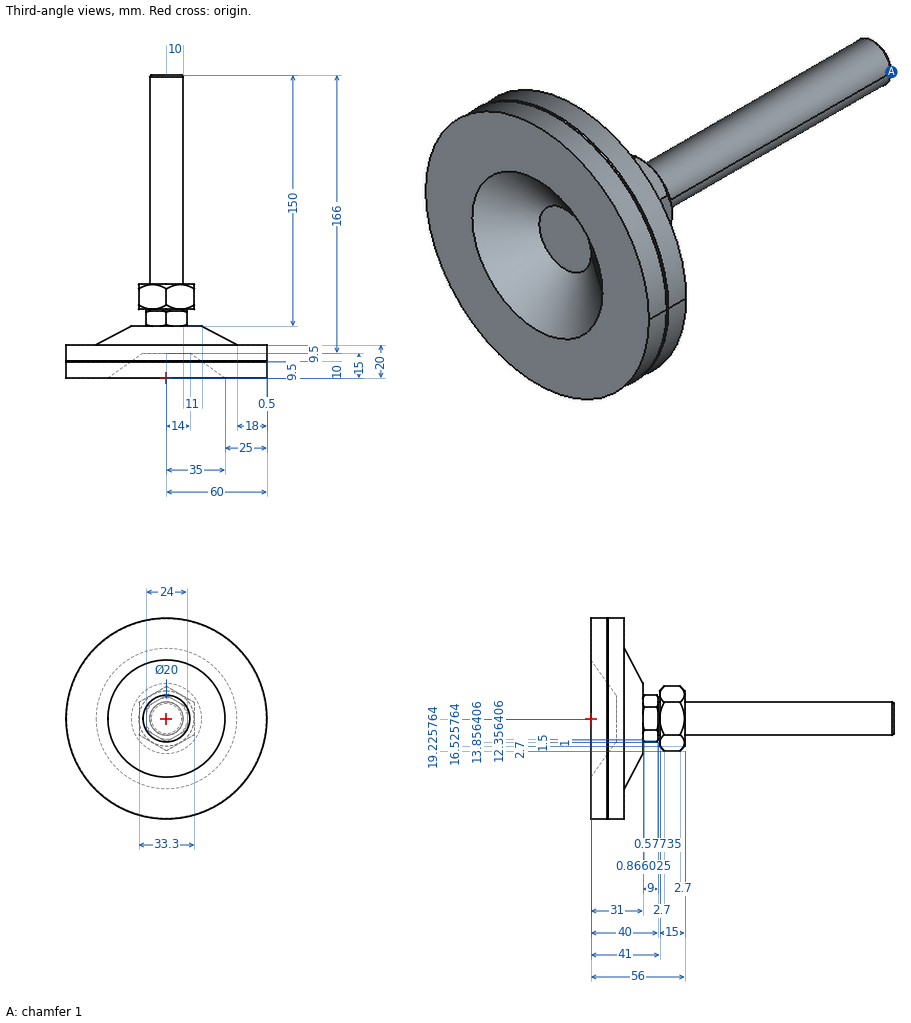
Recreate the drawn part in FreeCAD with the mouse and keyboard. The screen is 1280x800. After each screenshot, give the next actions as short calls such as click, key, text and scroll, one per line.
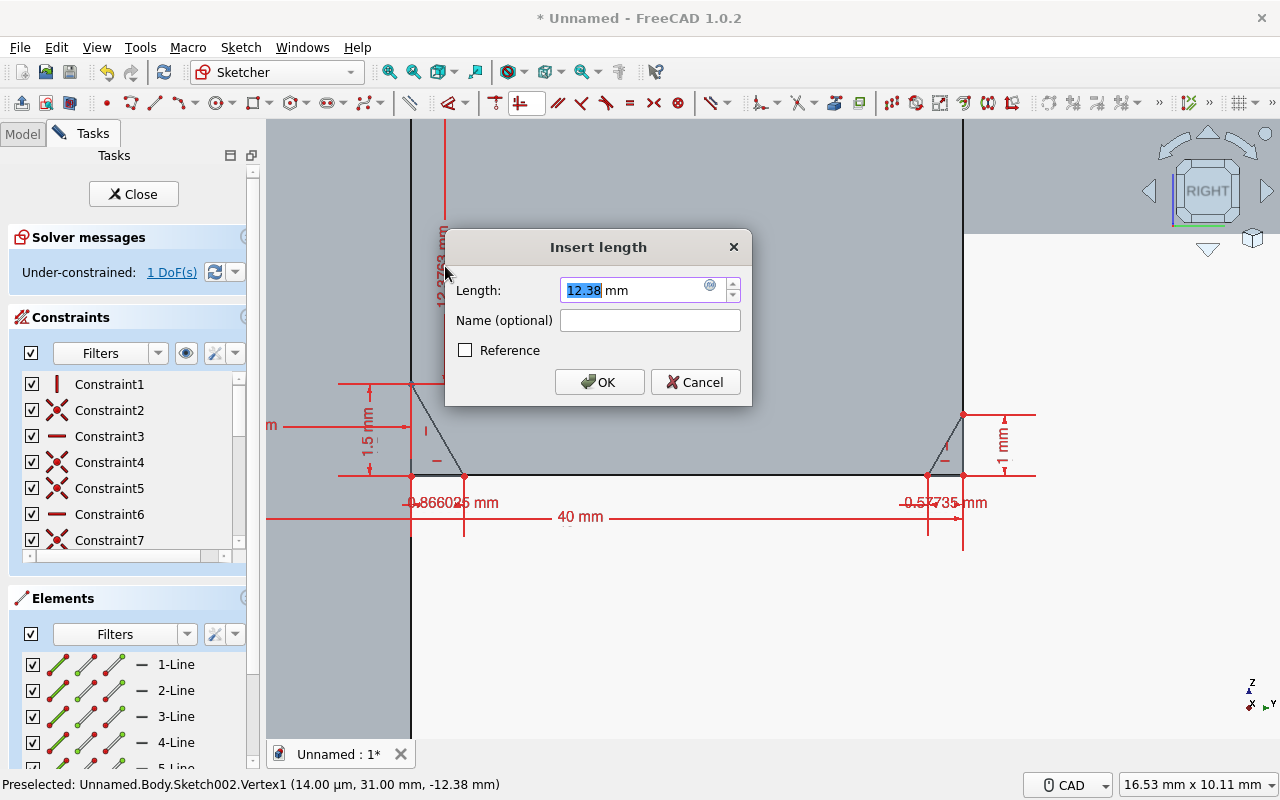
text(12.356406)
key(Return)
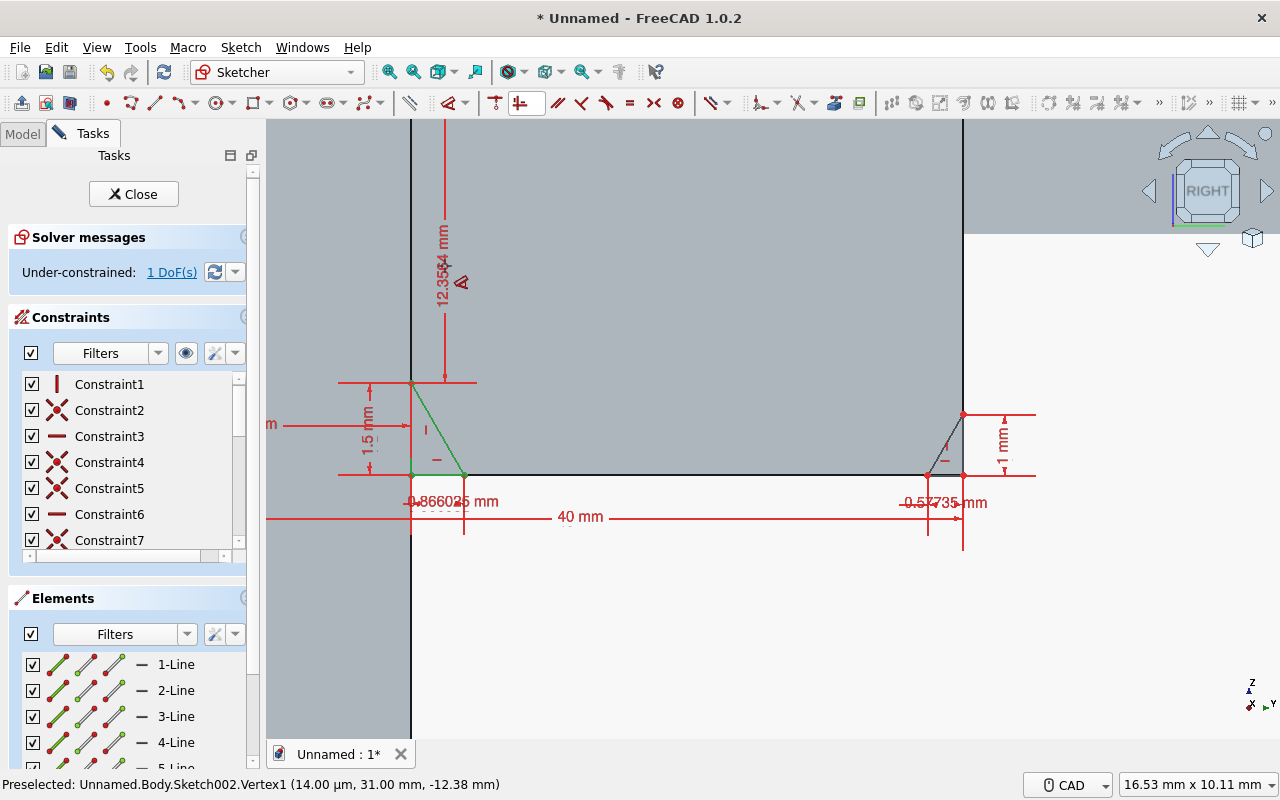
click(928, 476)
click(962, 311)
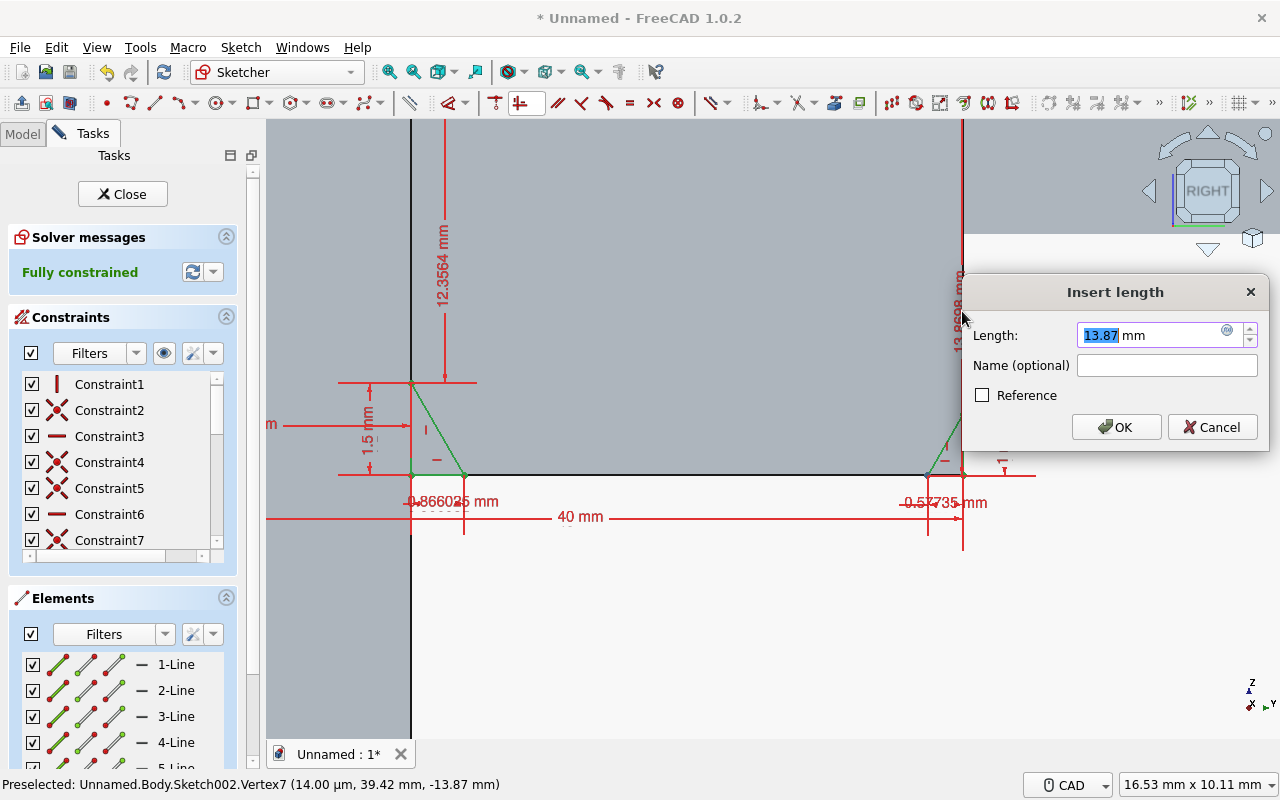
text(13.856406)
key(Return)
key(Escape)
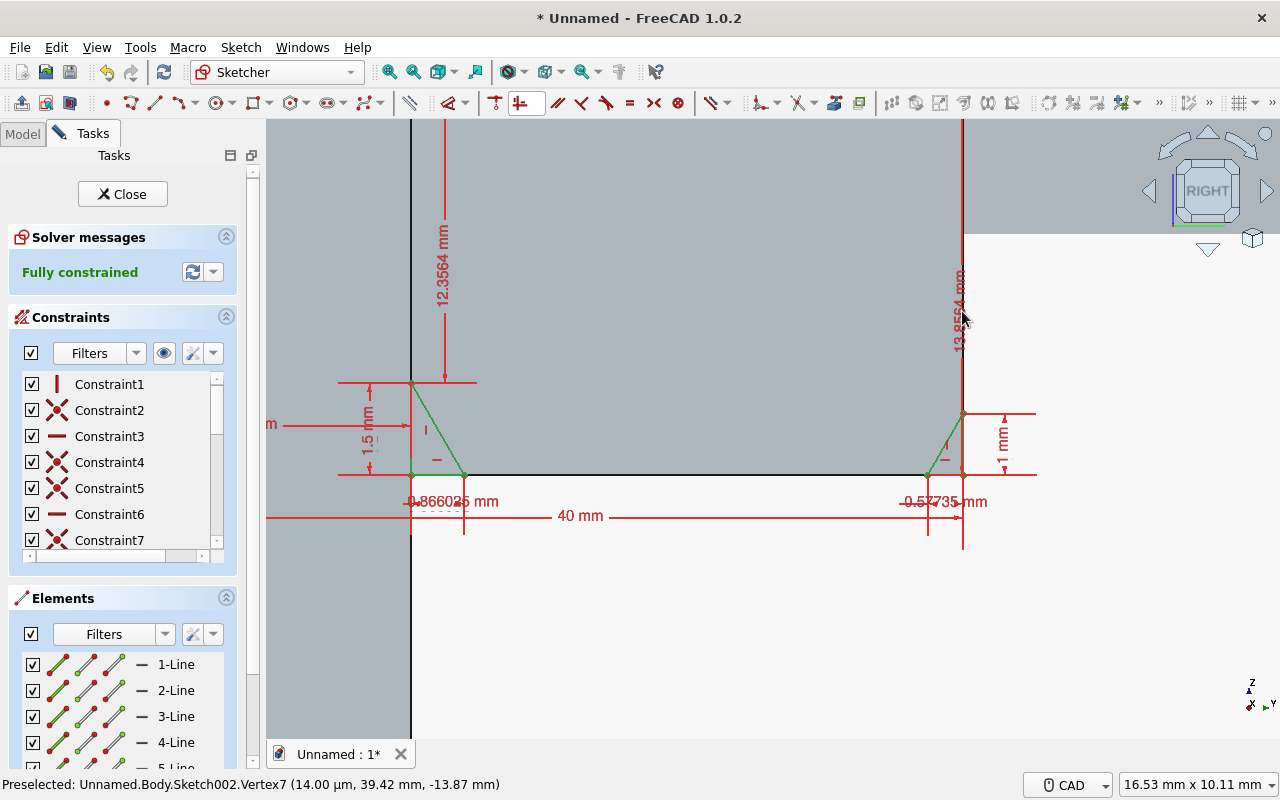
click(123, 194)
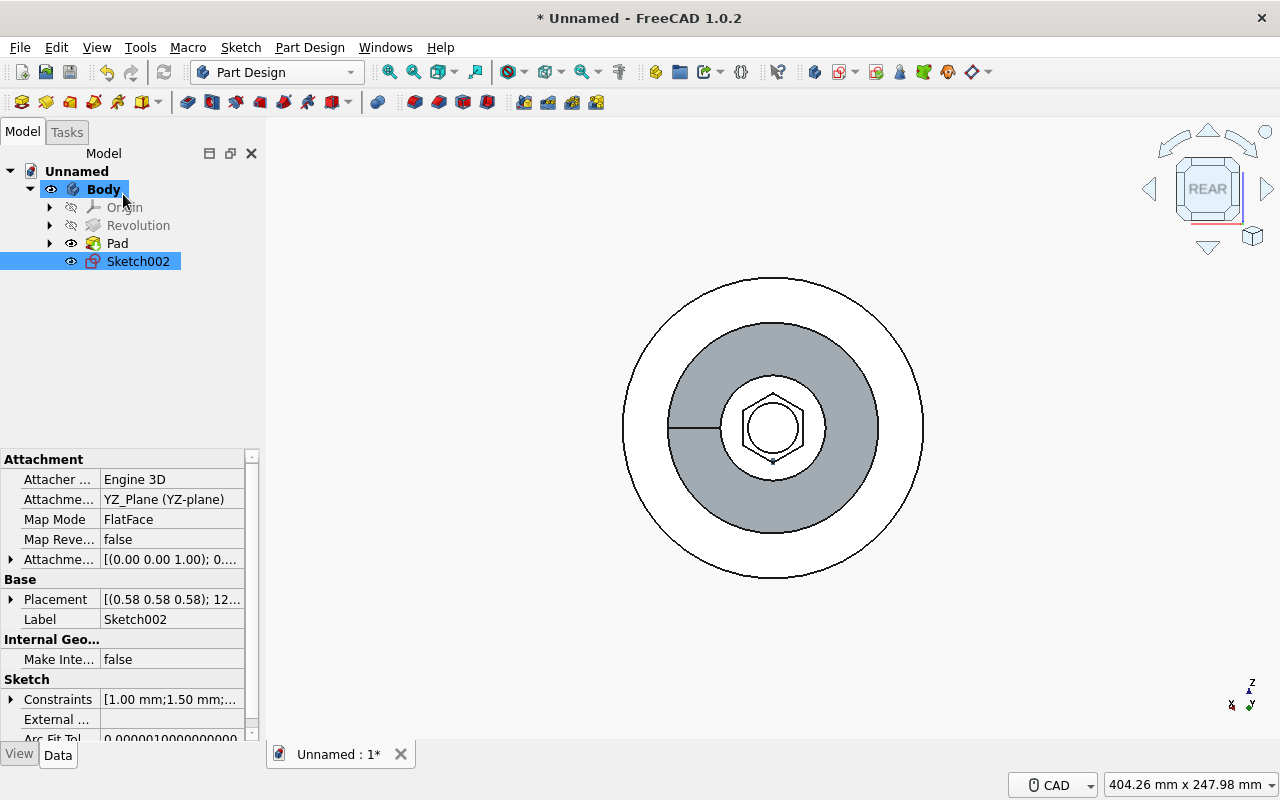
click(236, 102)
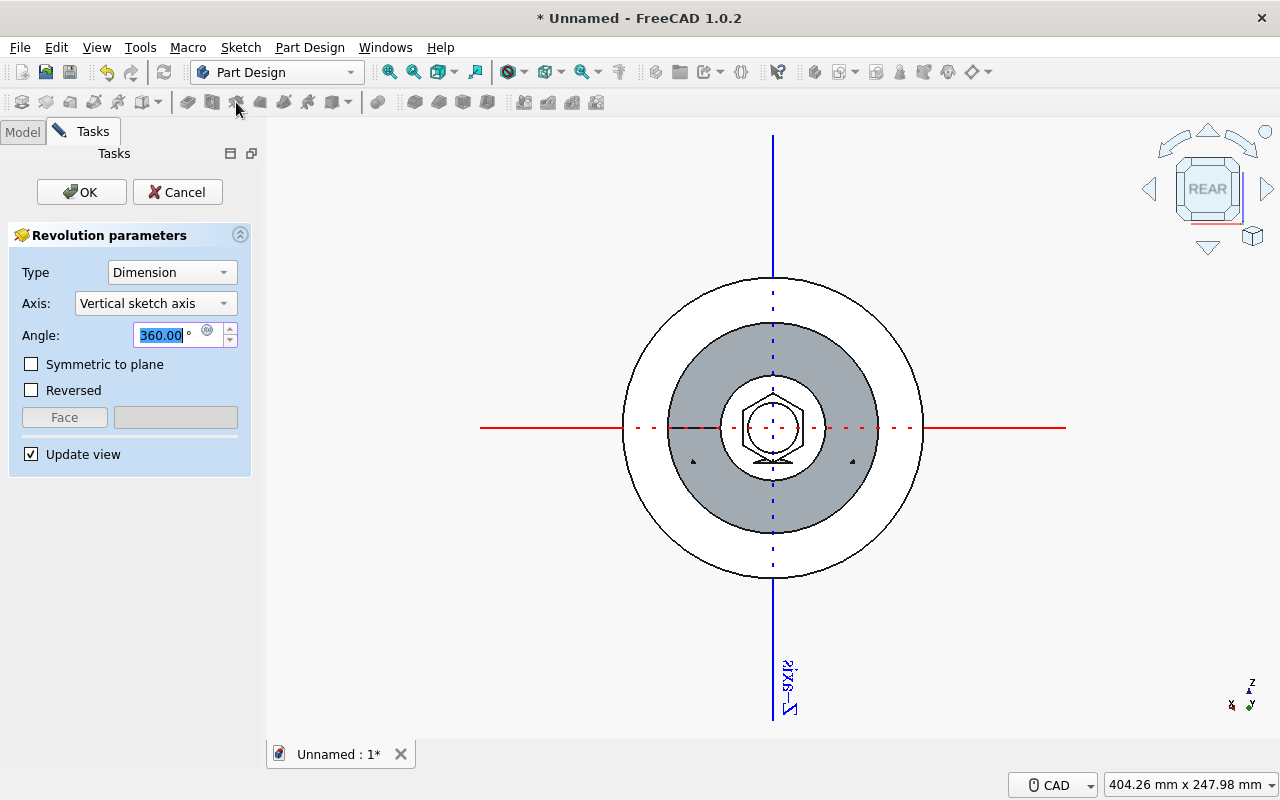
click(156, 304)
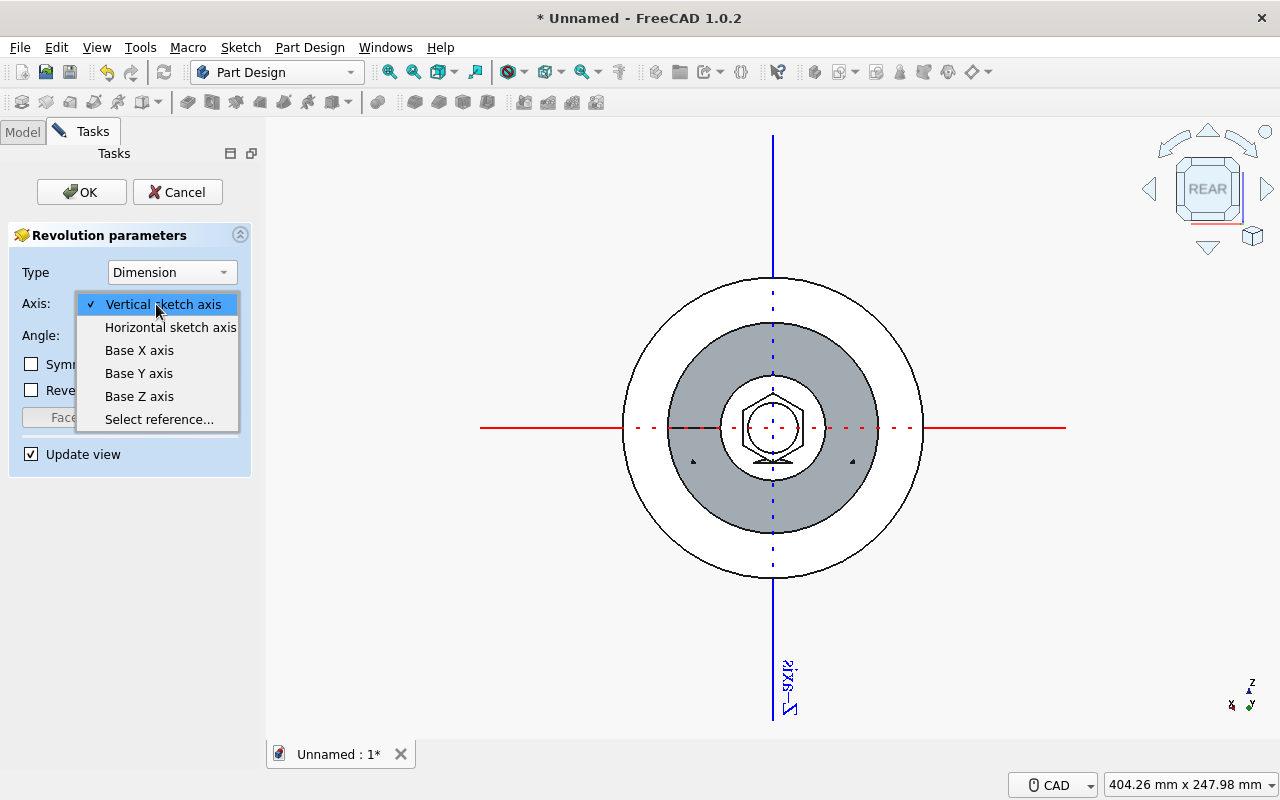
click(156, 328)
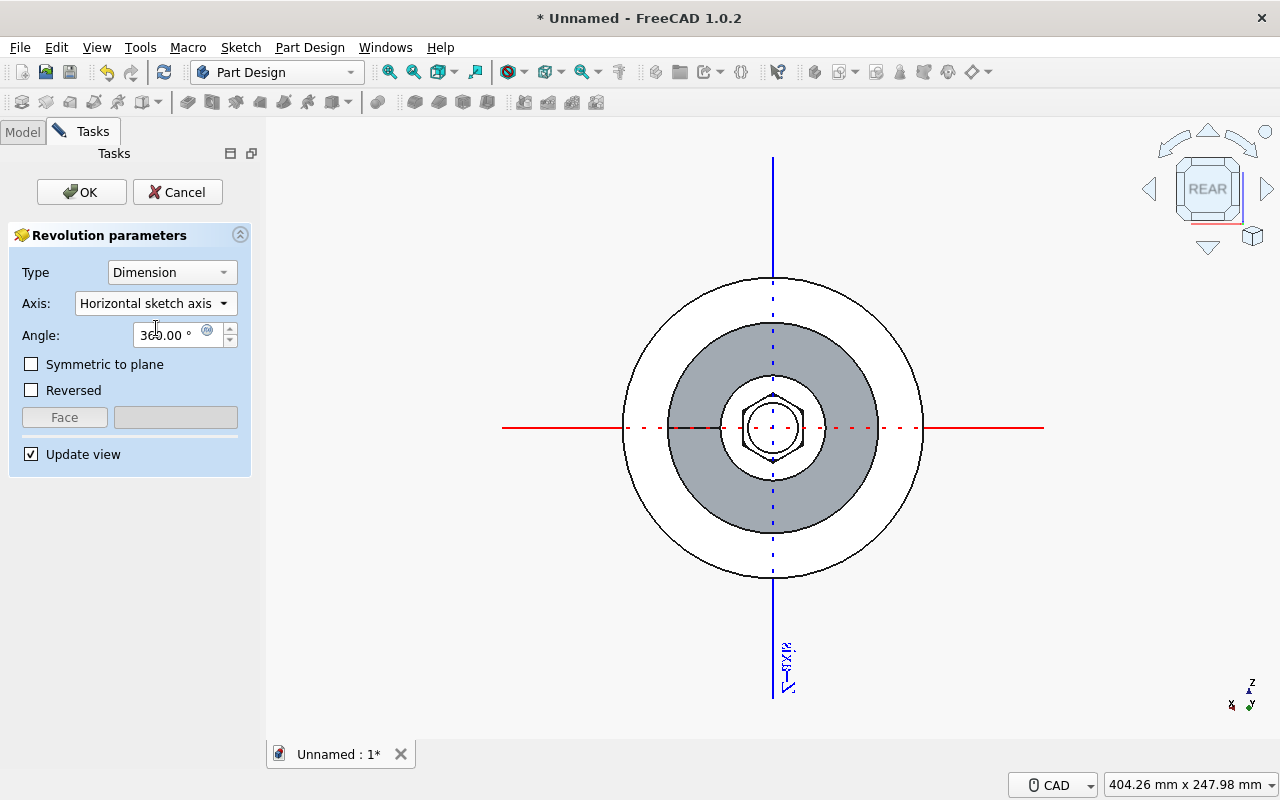
click(82, 192)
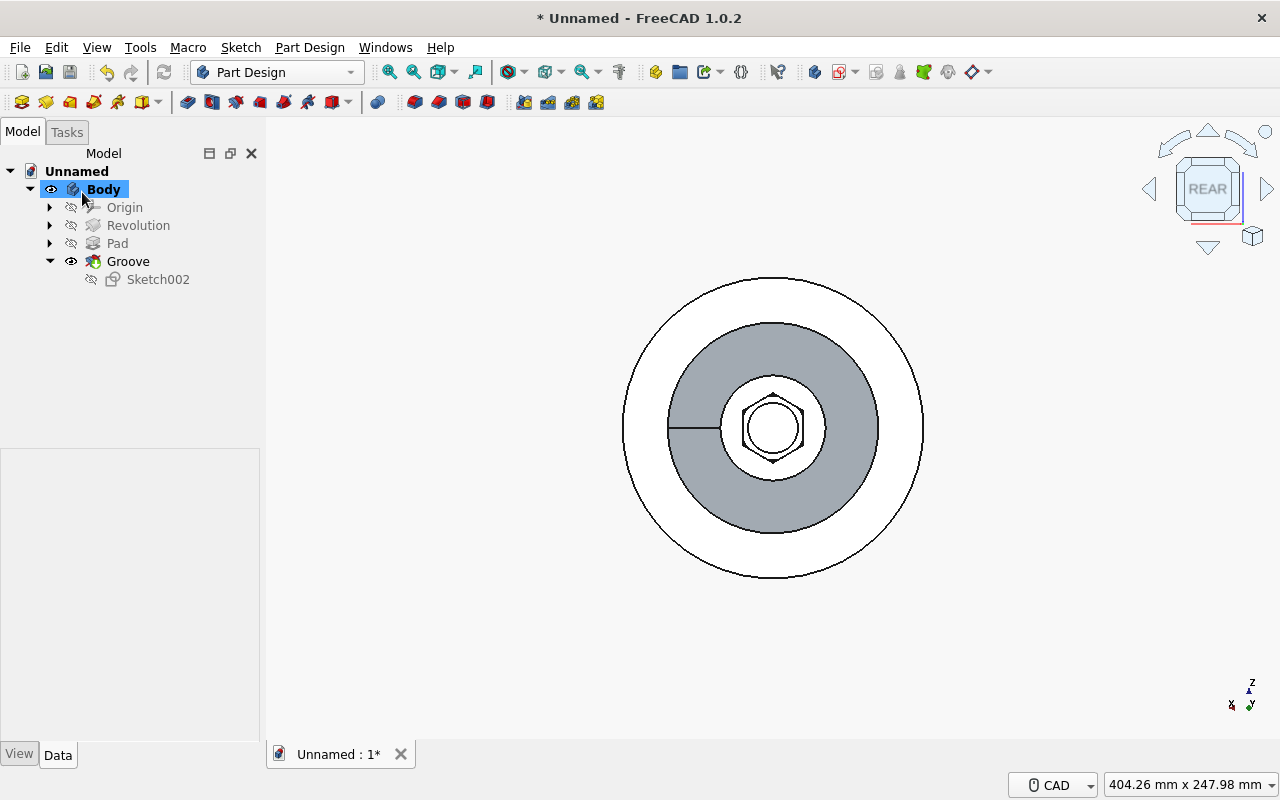
click(50, 207)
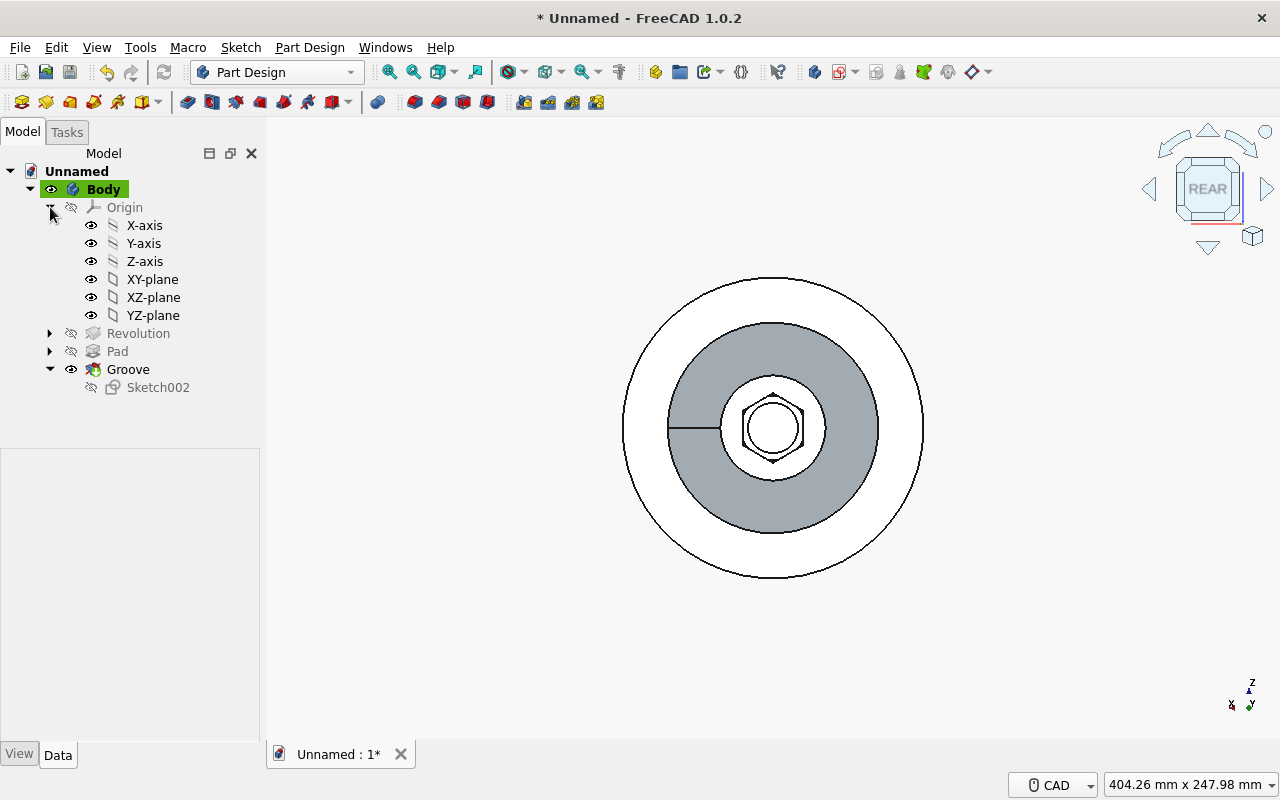
click(136, 297)